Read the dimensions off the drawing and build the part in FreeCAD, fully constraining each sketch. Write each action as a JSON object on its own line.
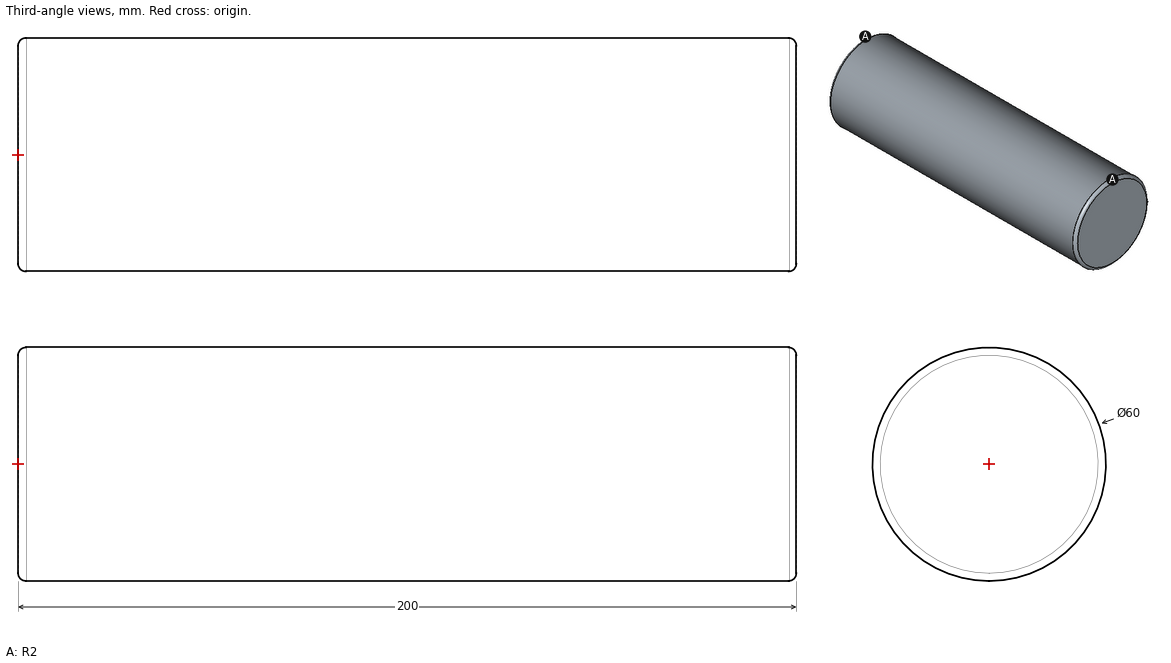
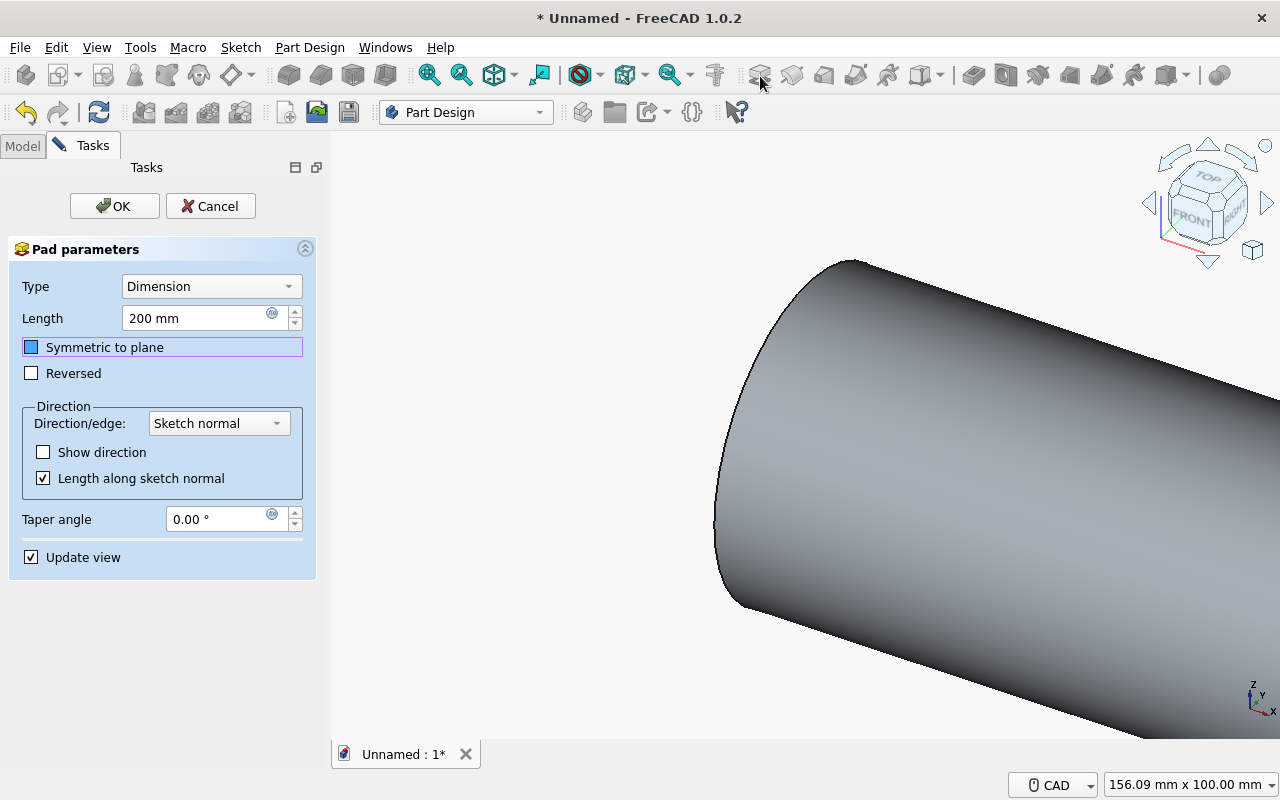
{"action": "left_click", "coordinate": [115, 206]}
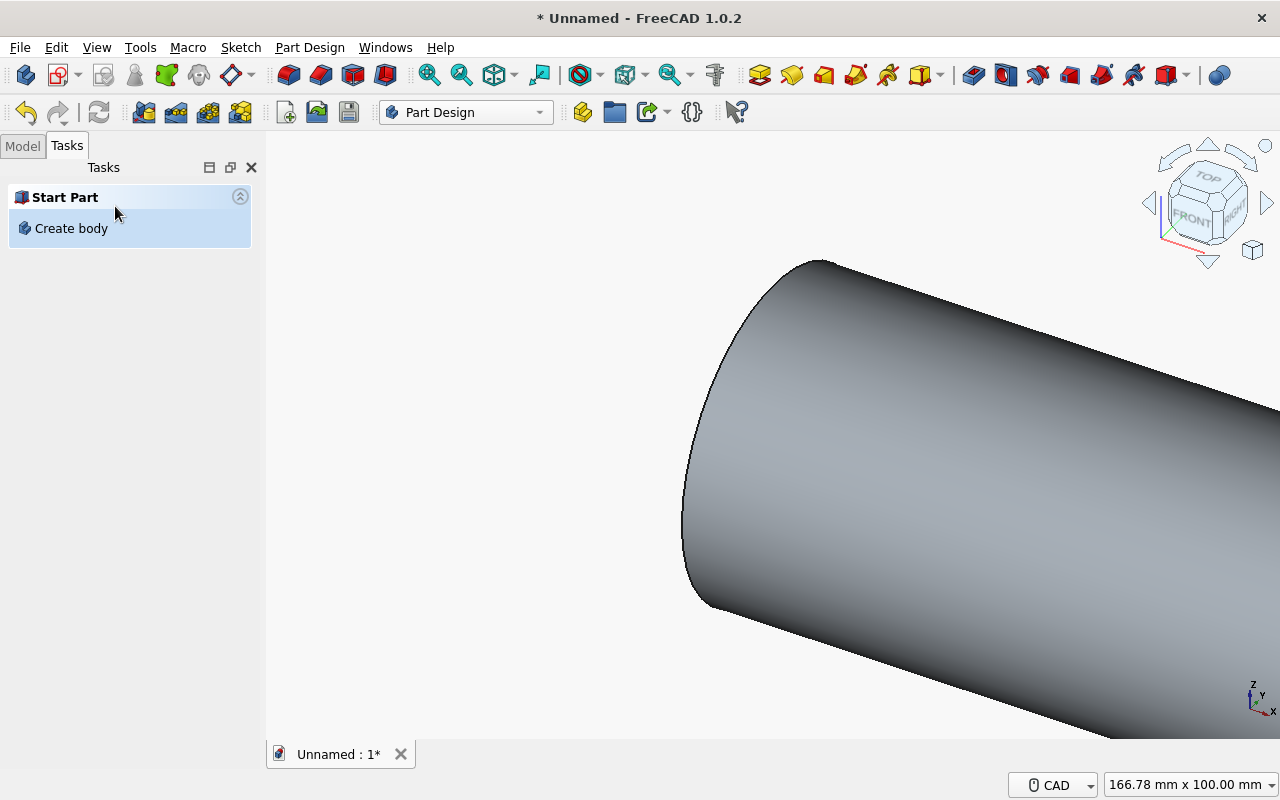
{"action": "key", "text": "v f"}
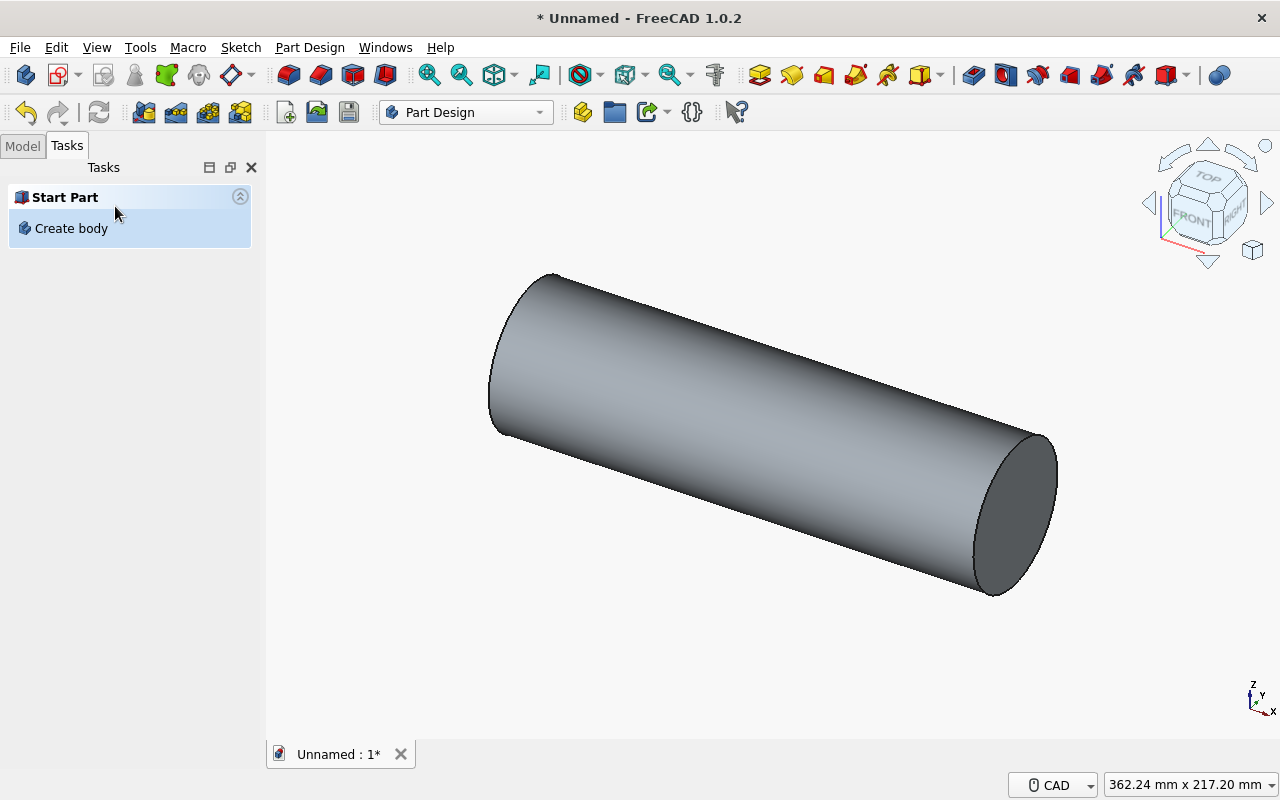
{"action": "left_click", "coordinate": [973, 556]}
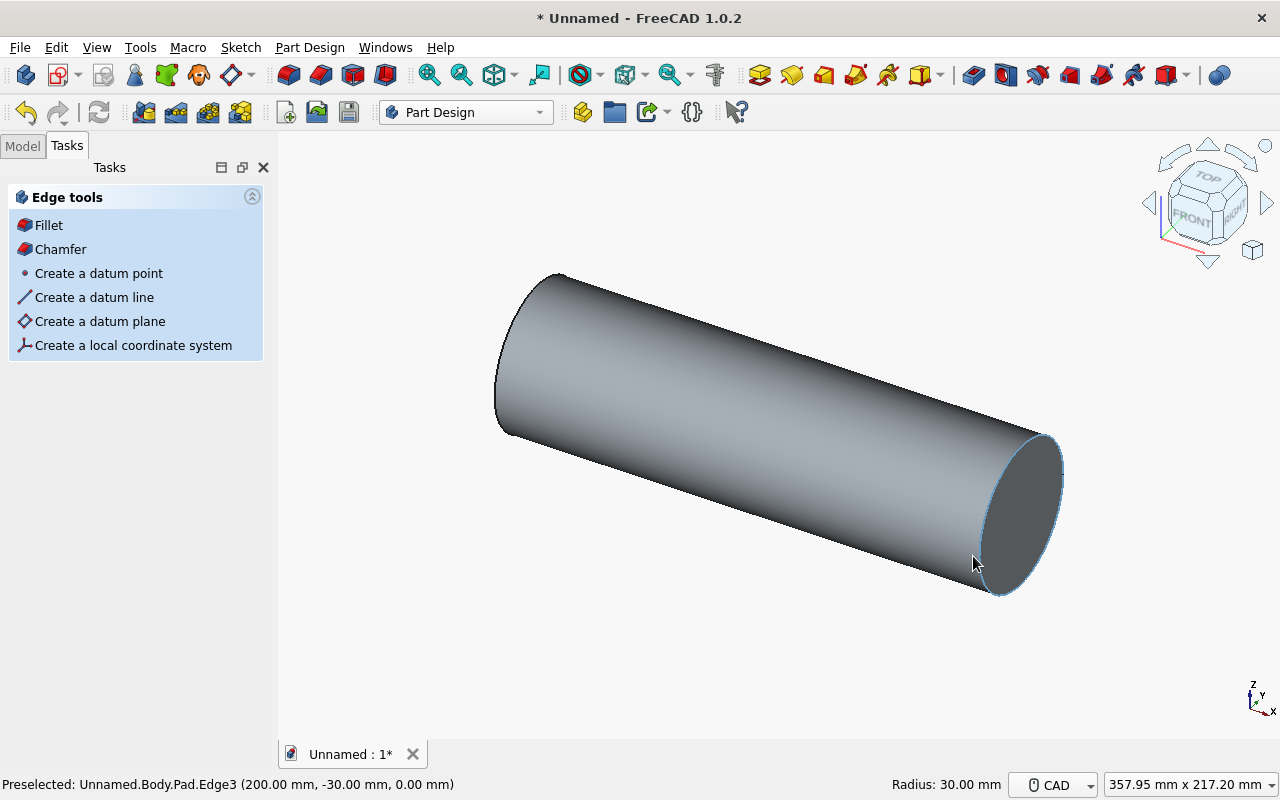
{"action": "key", "text": "0"}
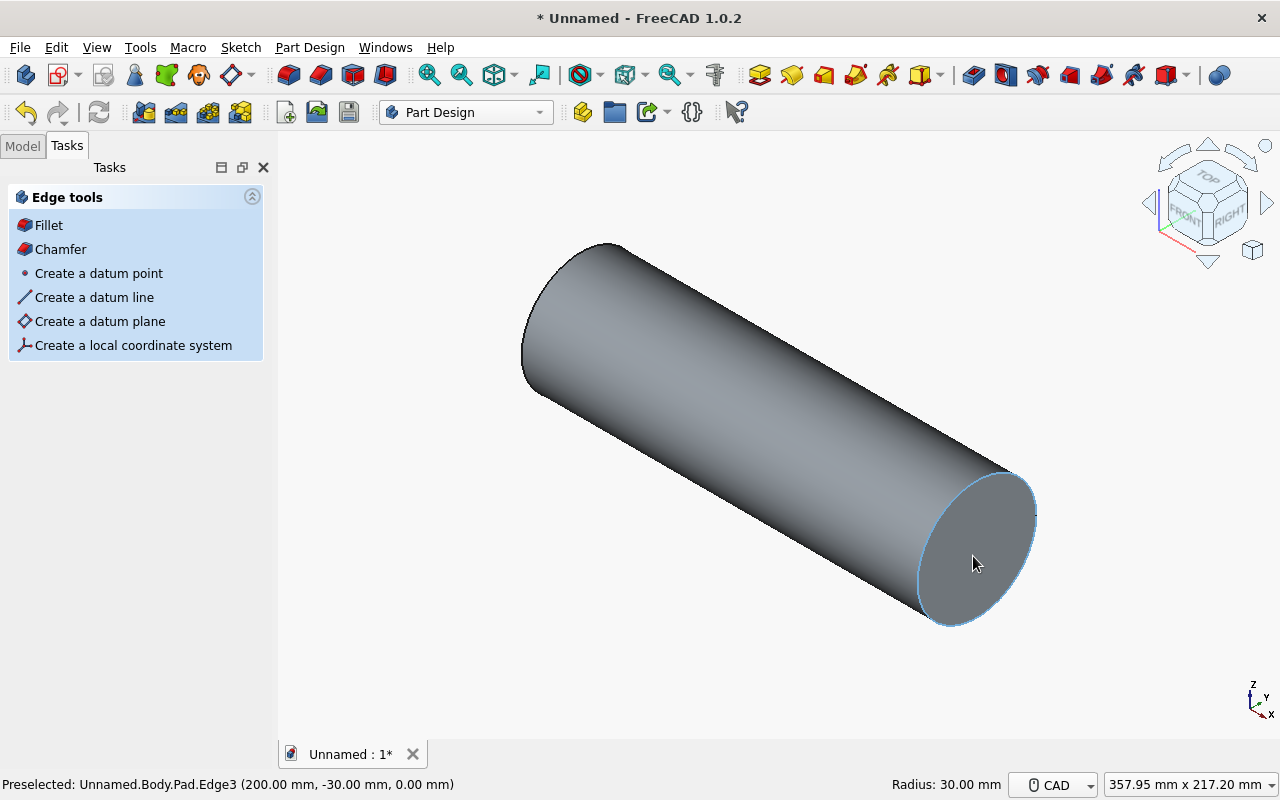
{"action": "key", "text": "2"}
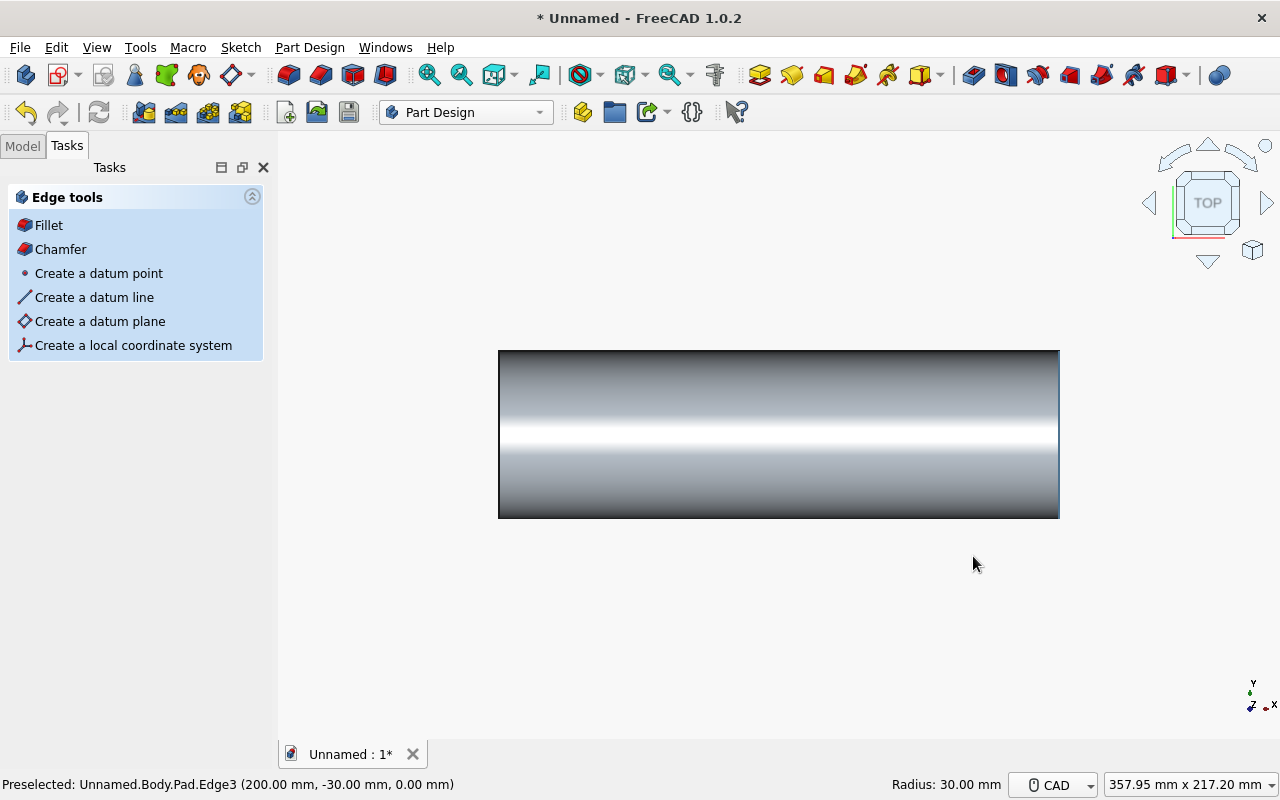
{"action": "left_click", "coordinate": [499, 502], "text": "ctrl"}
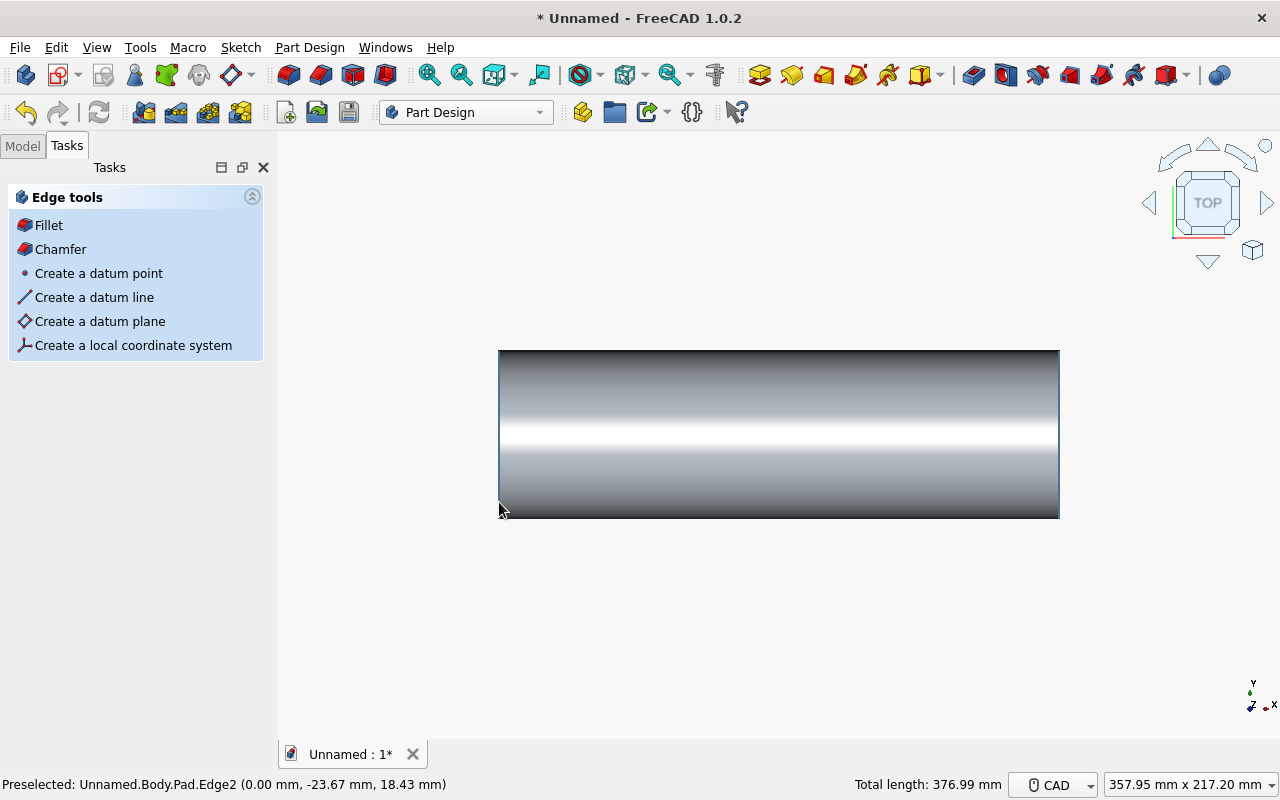
{"action": "left_click", "coordinate": [290, 76]}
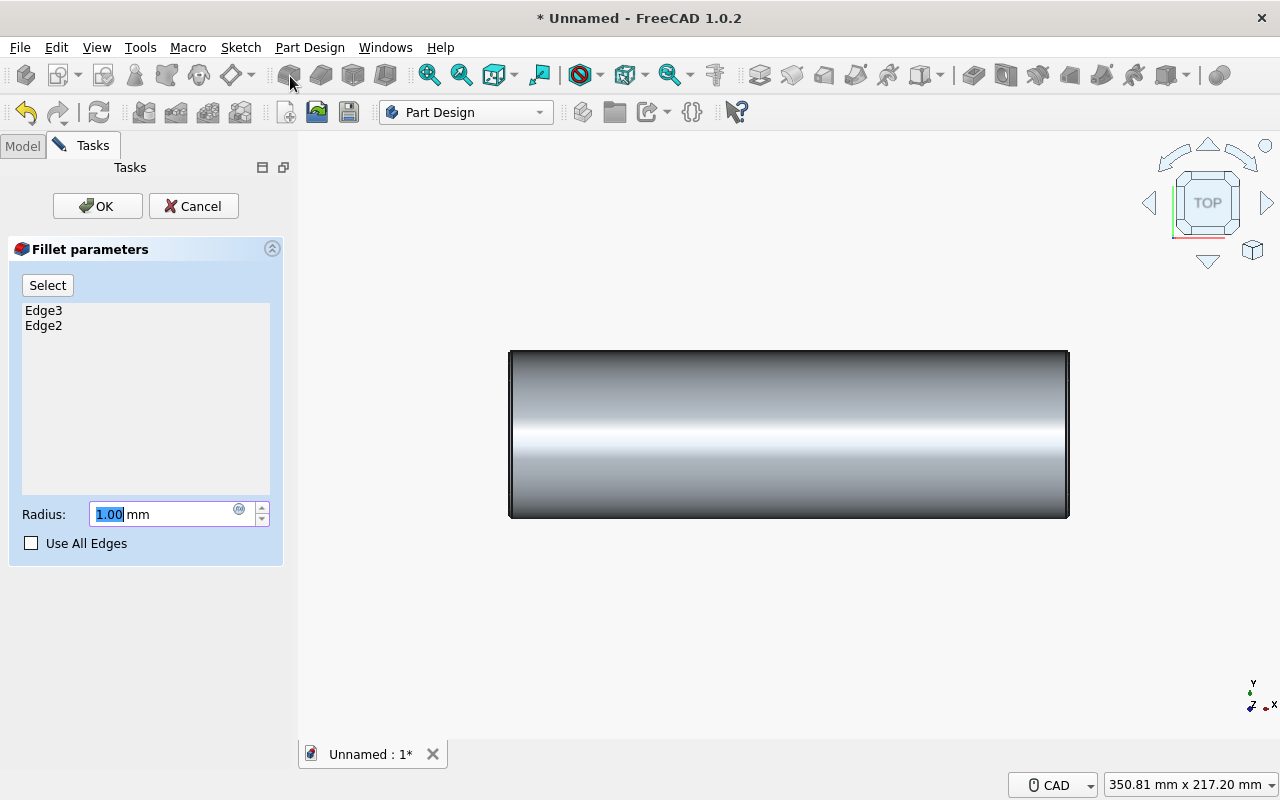
{"action": "type", "text": "2"}
{"action": "key", "text": "Tab"}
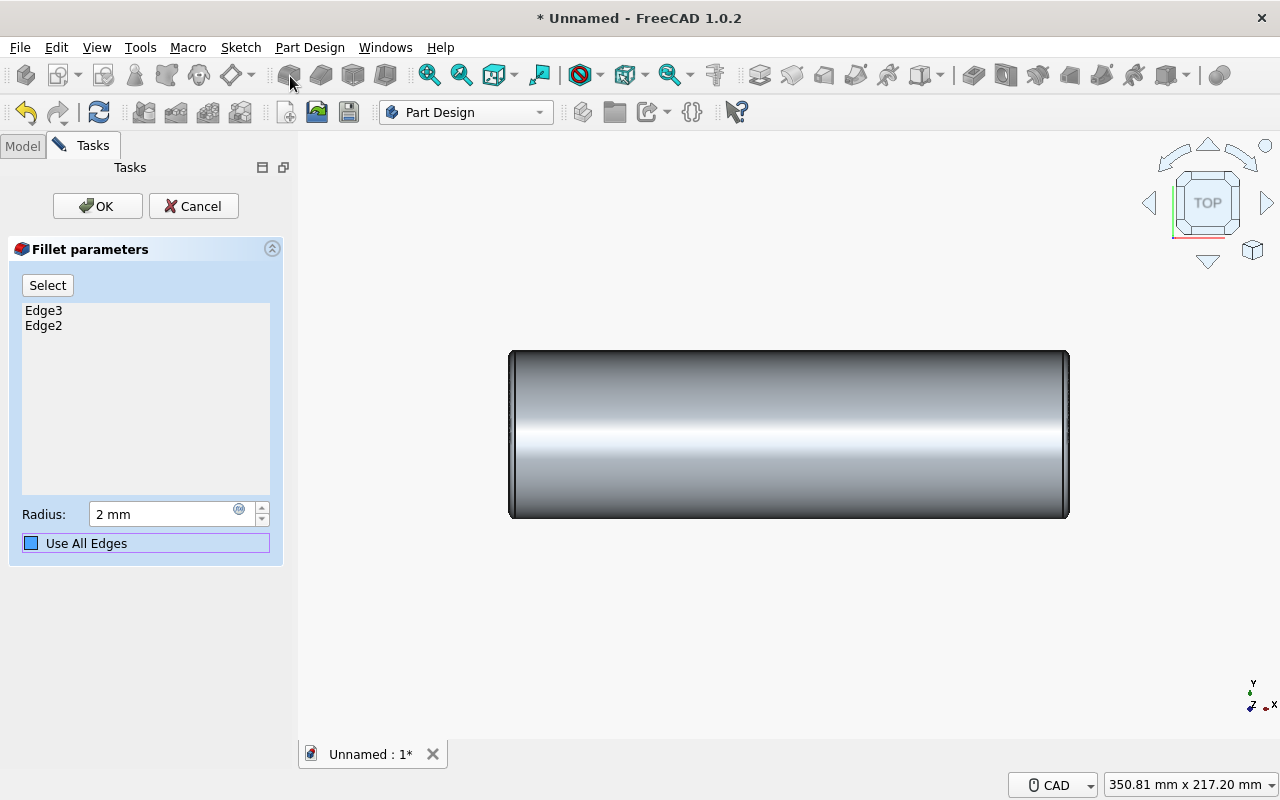
{"action": "left_click", "coordinate": [98, 206]}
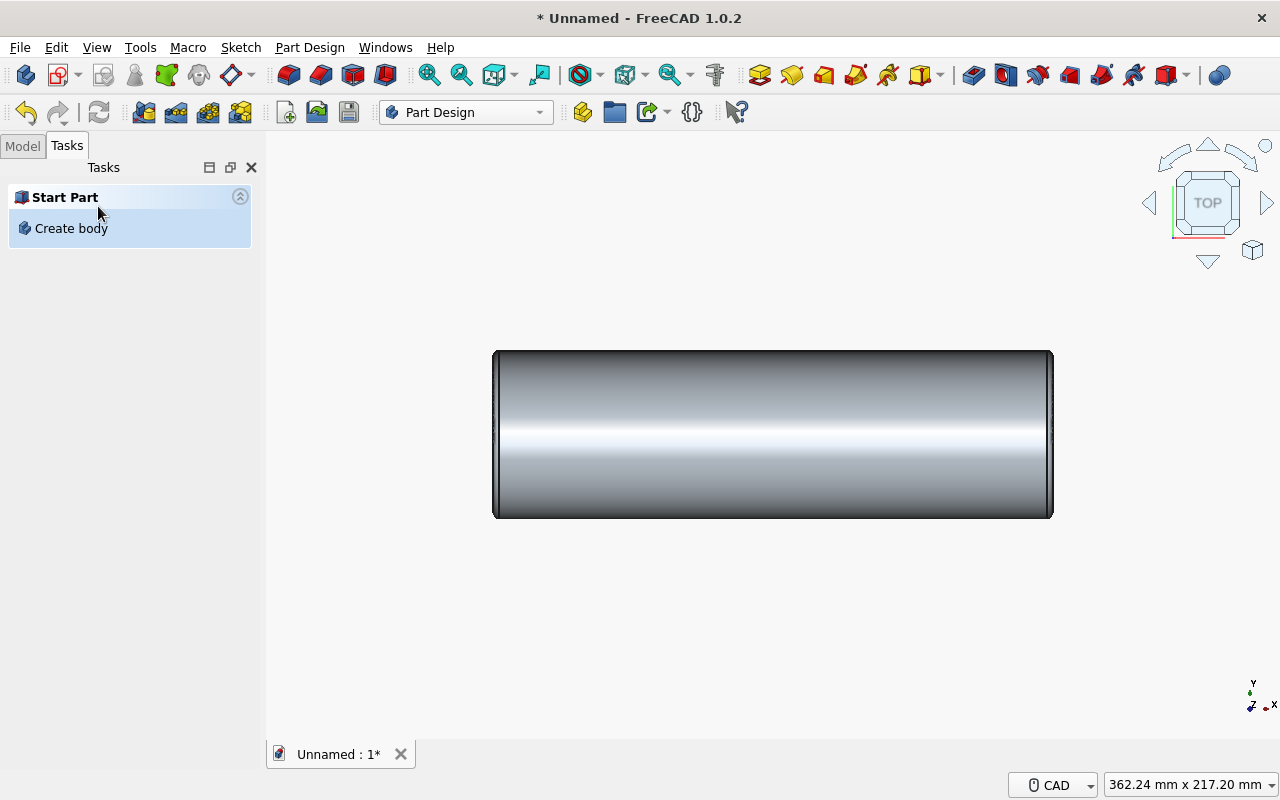
{"action": "key", "text": "0"}